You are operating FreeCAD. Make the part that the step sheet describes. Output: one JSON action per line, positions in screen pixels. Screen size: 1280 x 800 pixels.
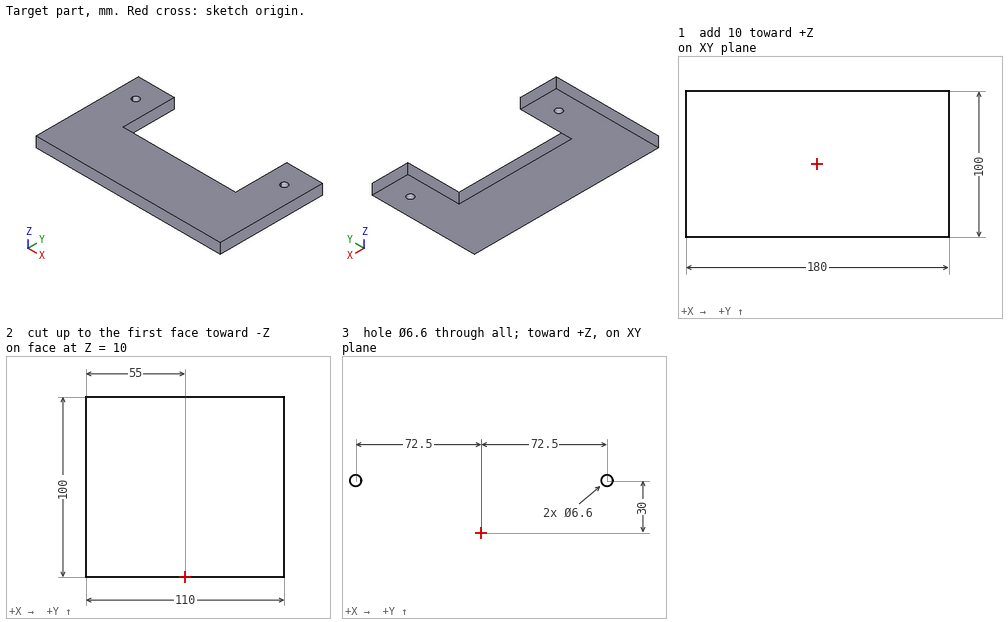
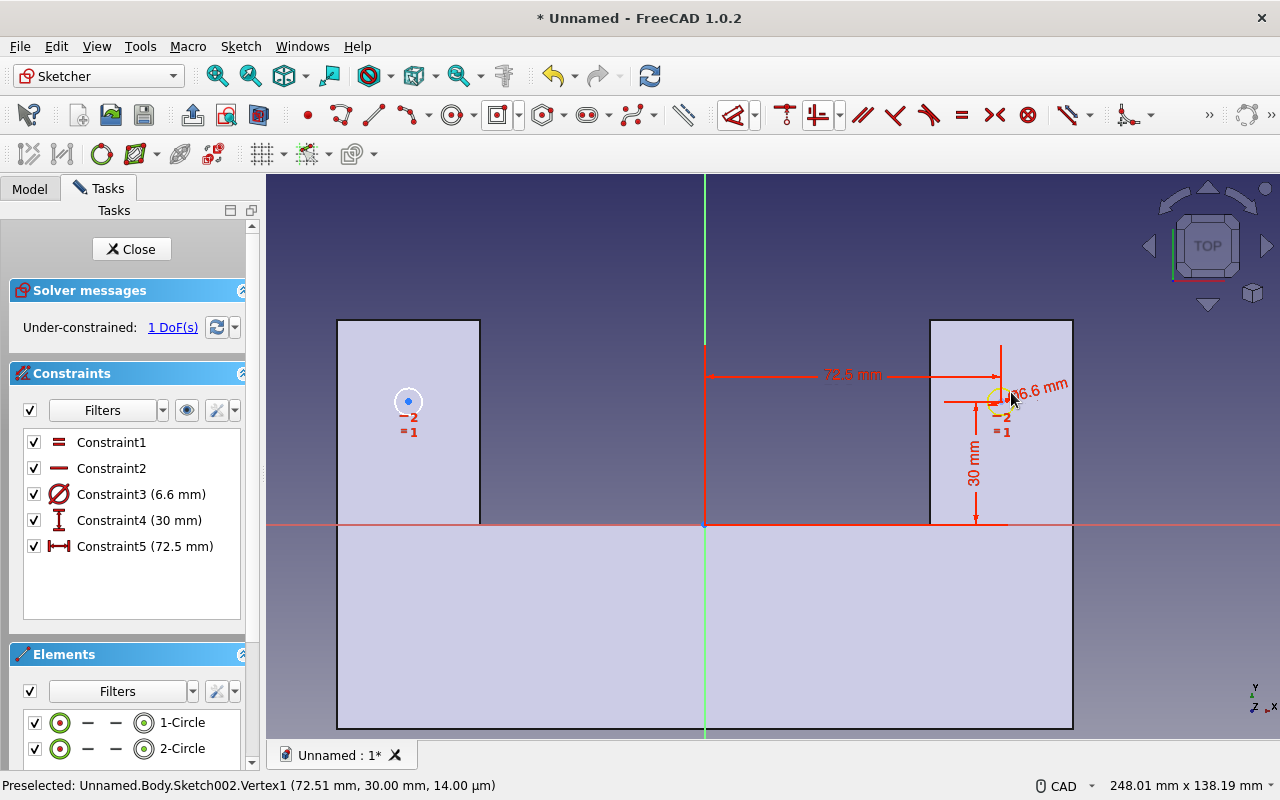
{"action": "left_click", "coordinate": [409, 402]}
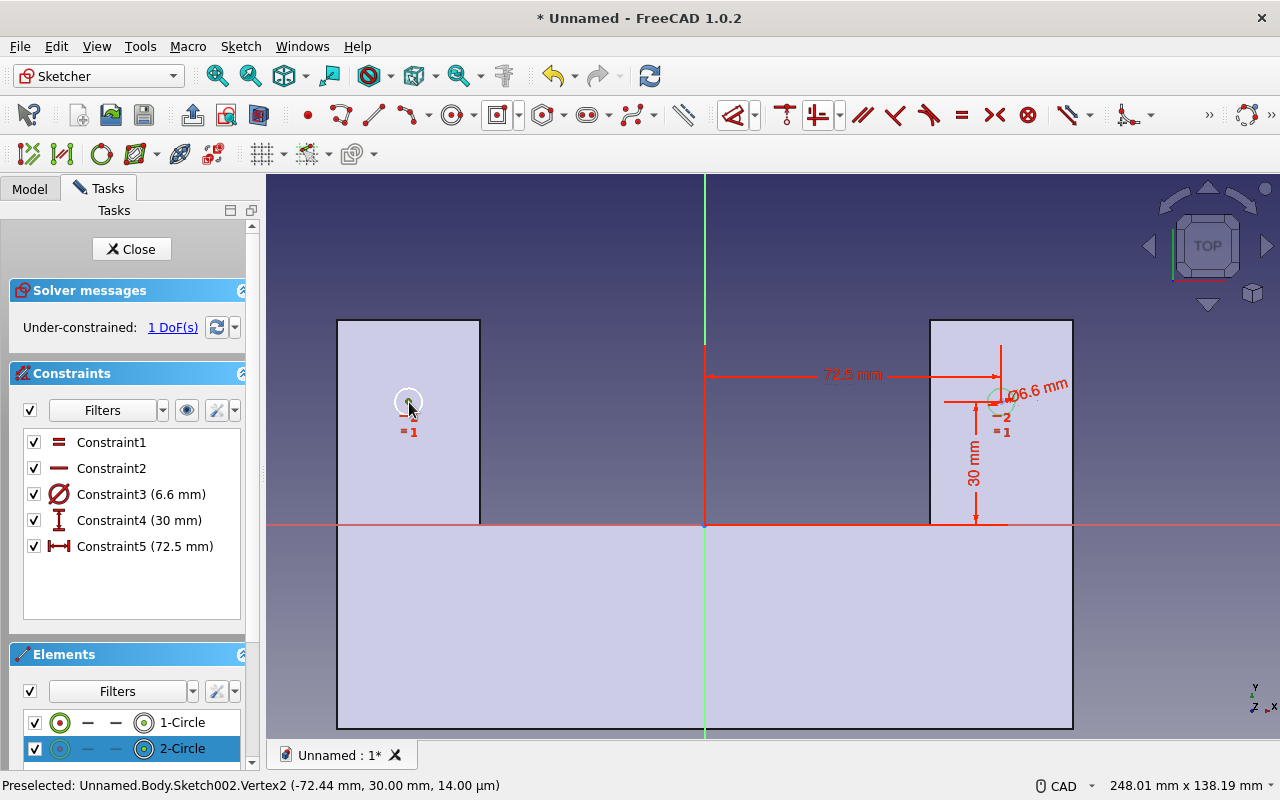
{"action": "left_click", "coordinate": [754, 116]}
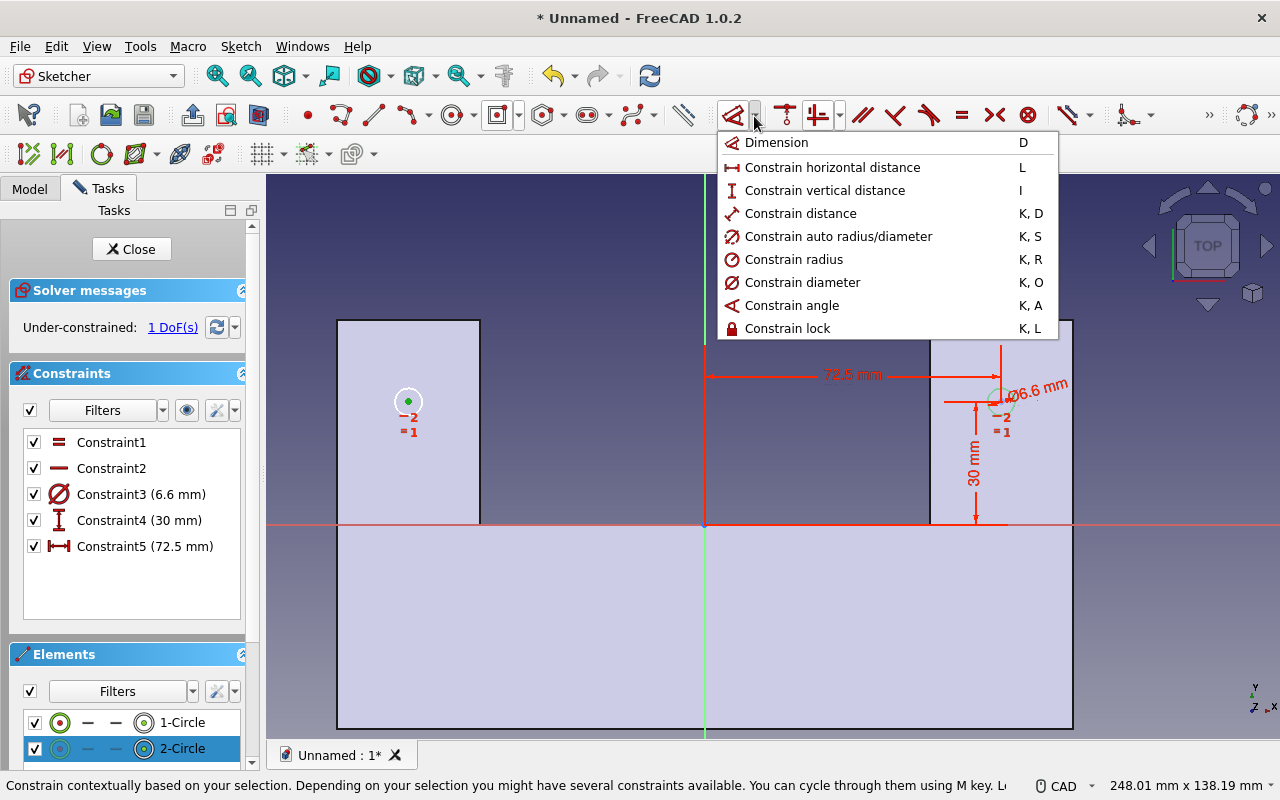
{"action": "left_click", "coordinate": [888, 168]}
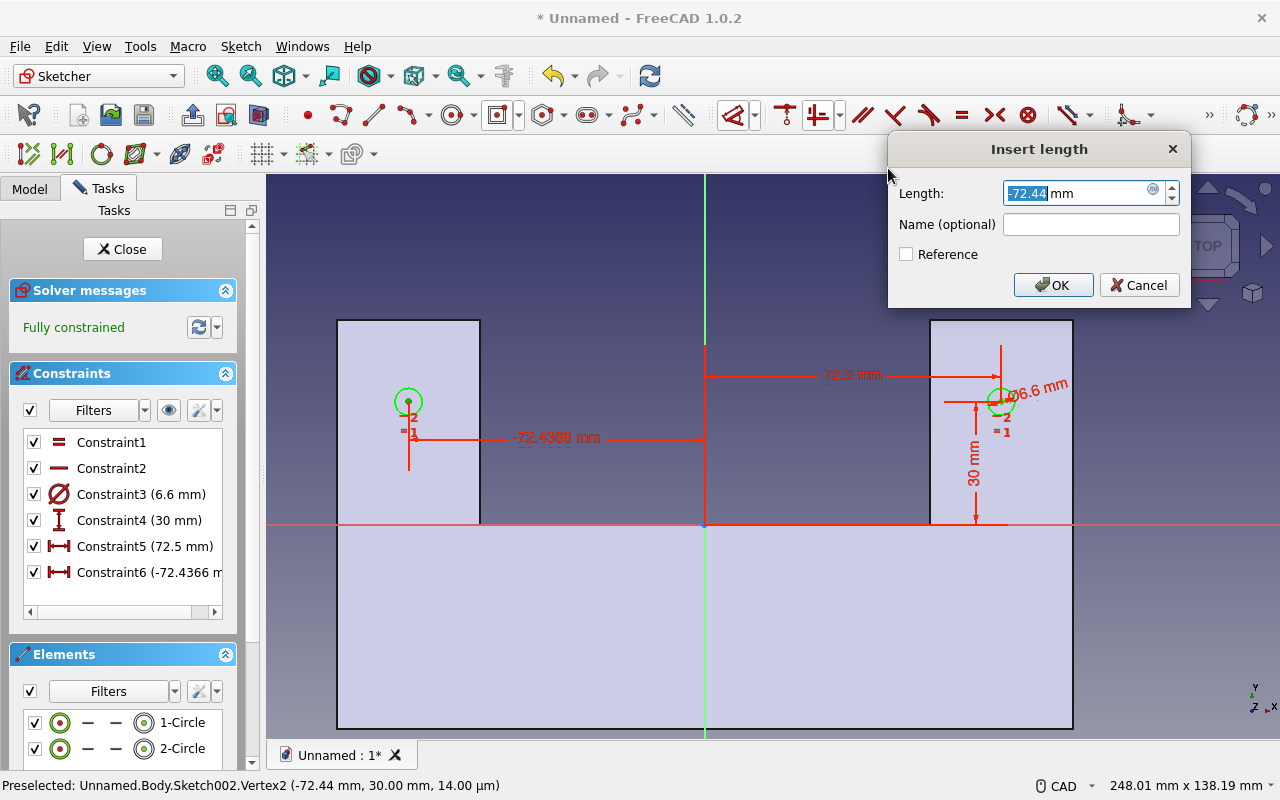
{"action": "type", "text": "-72.5"}
{"action": "key", "text": "Return"}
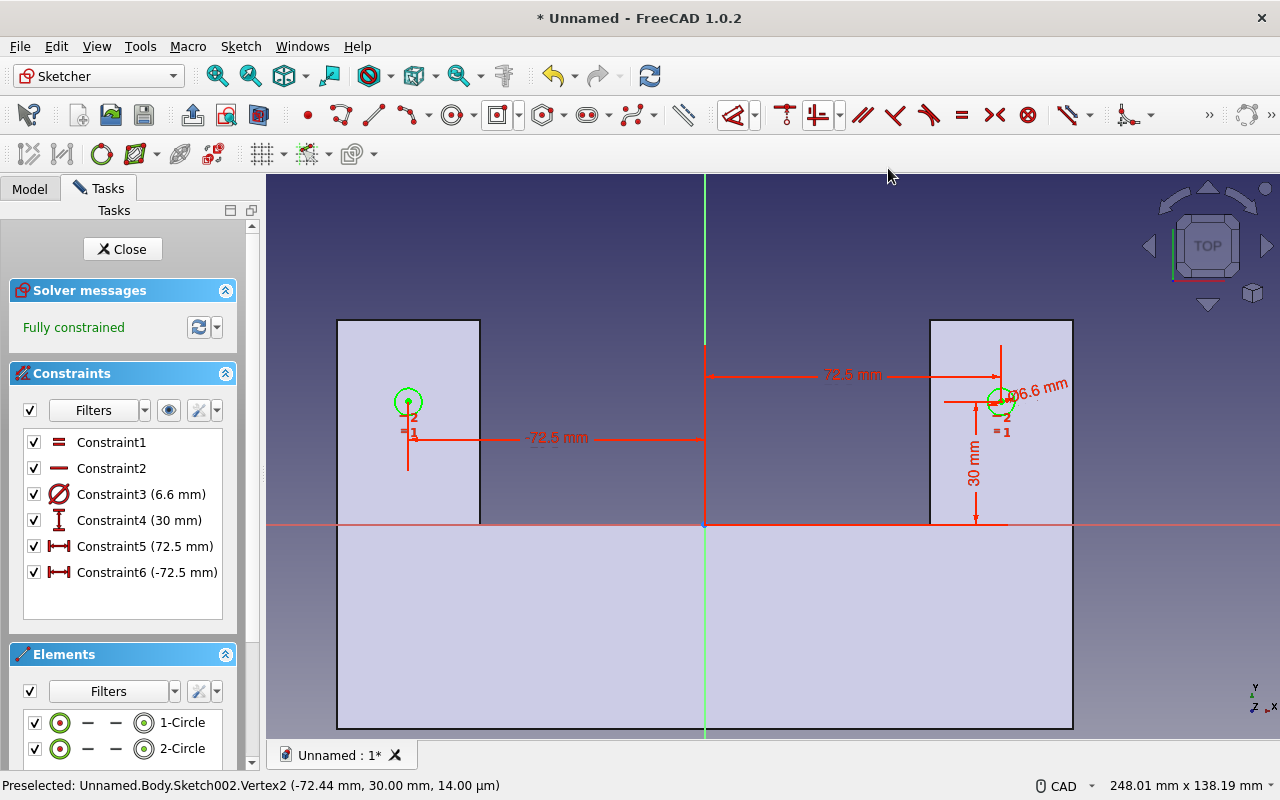
{"action": "left_click", "coordinate": [123, 249]}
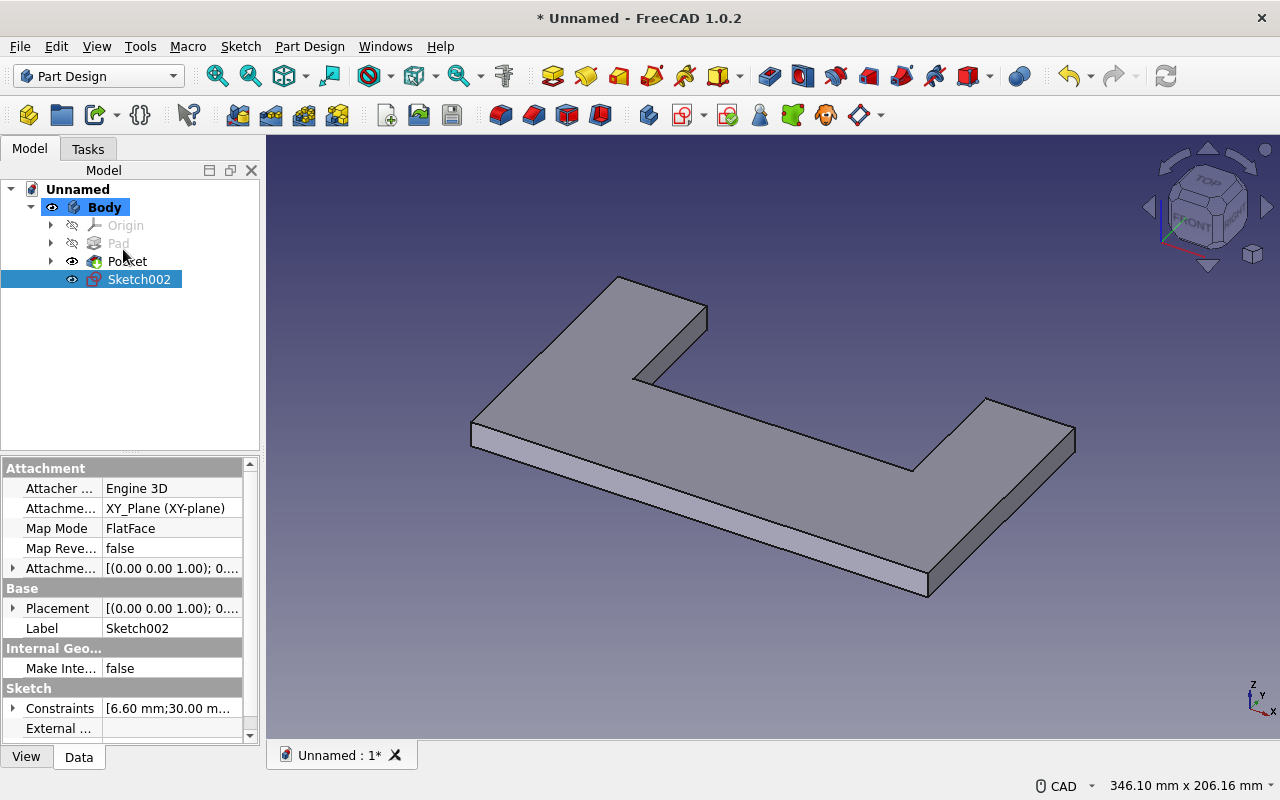
{"action": "left_click", "coordinate": [803, 76]}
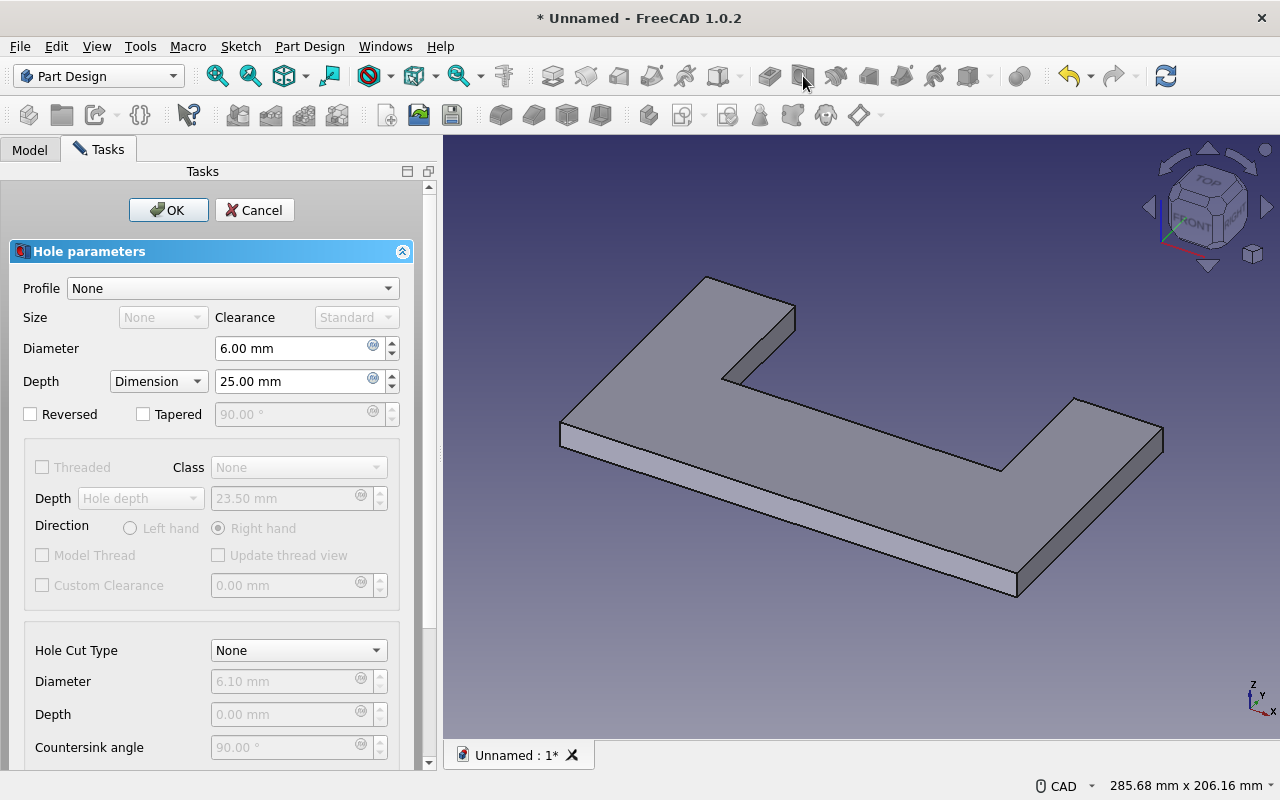
{"action": "triple_click", "coordinate": [300, 348]}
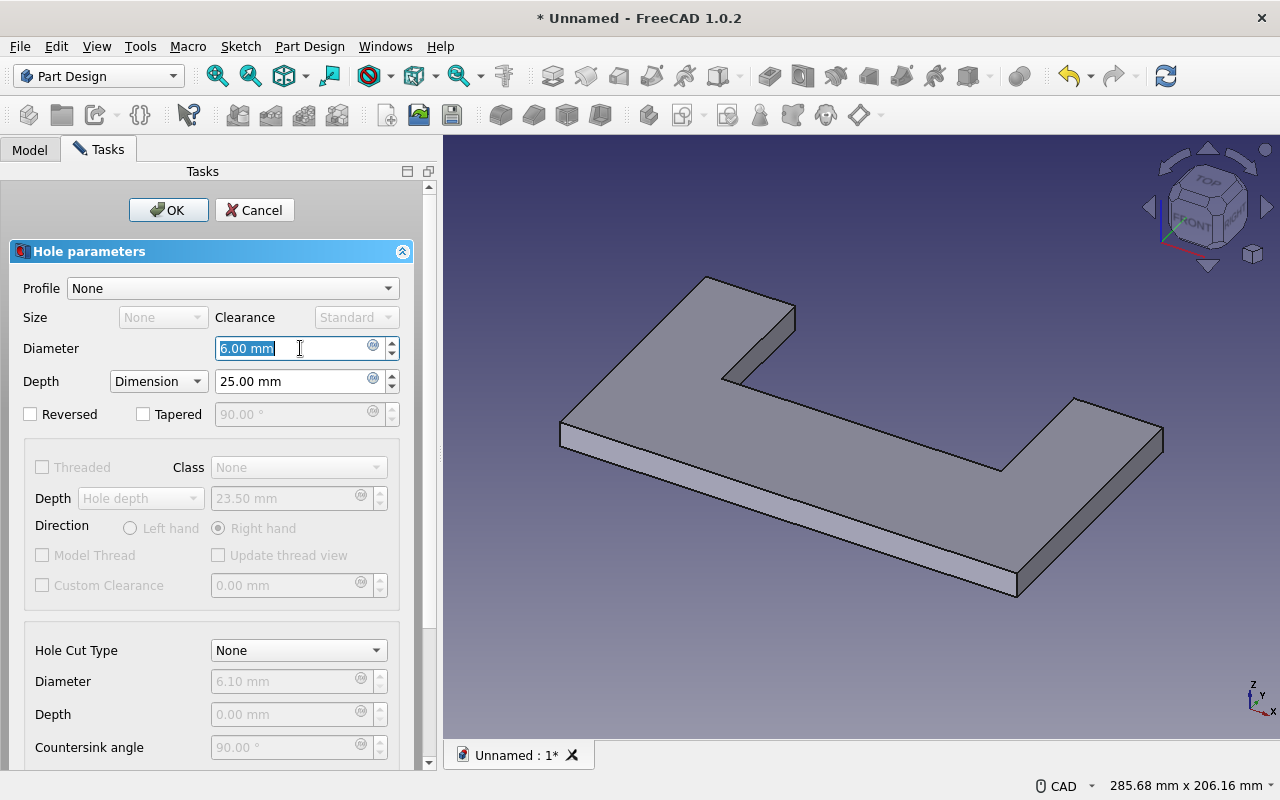
{"action": "type", "text": "6.6"}
{"action": "key", "text": "Tab"}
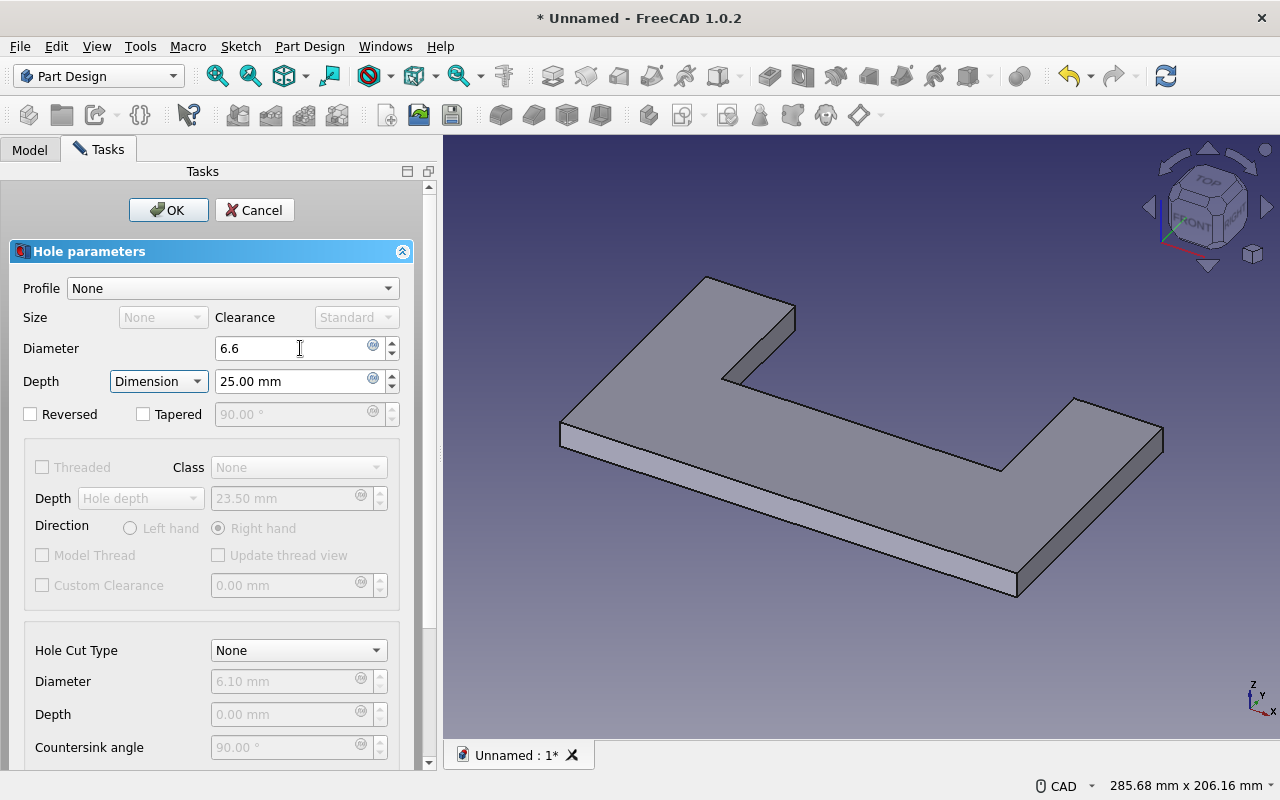
{"action": "left_click", "coordinate": [160, 382]}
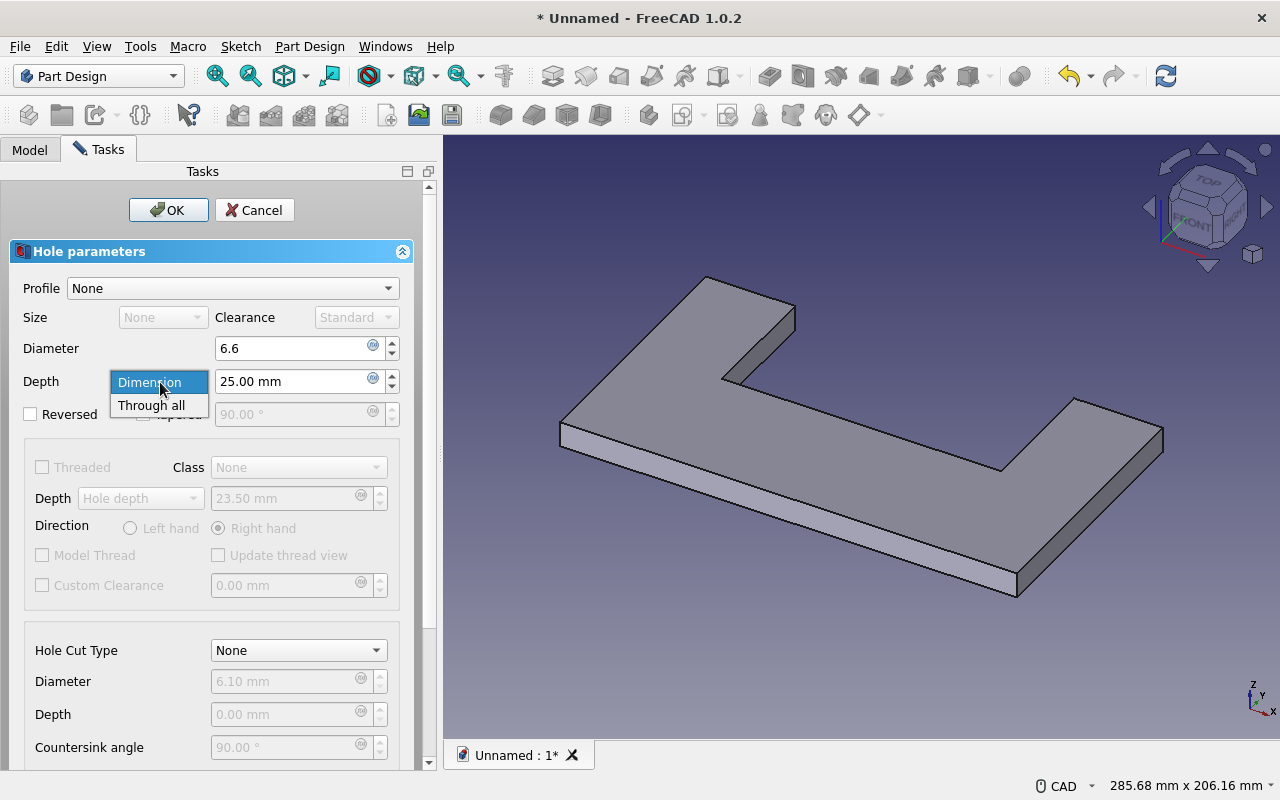
{"action": "left_click", "coordinate": [158, 406]}